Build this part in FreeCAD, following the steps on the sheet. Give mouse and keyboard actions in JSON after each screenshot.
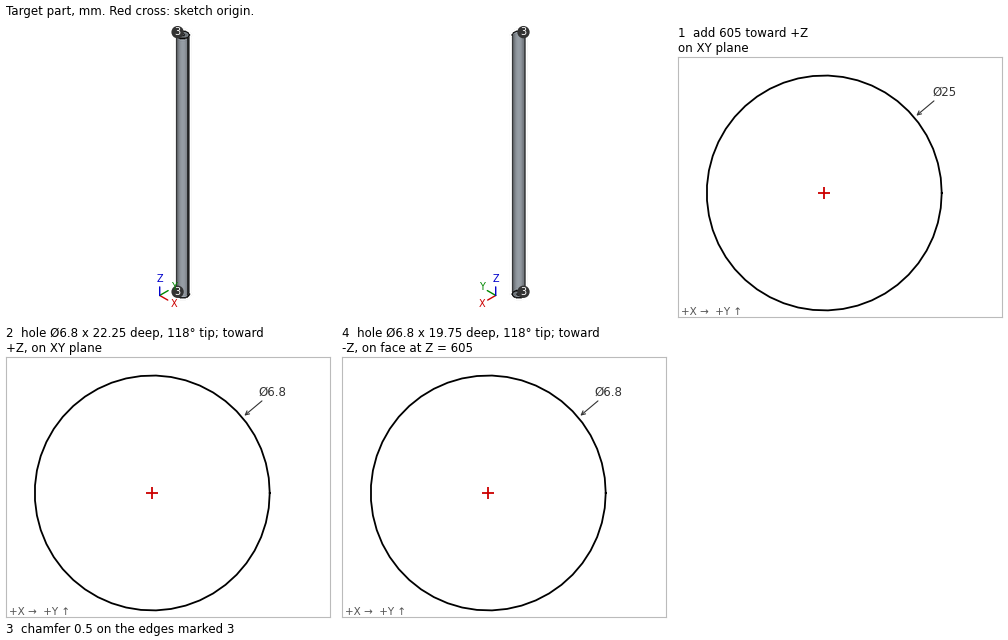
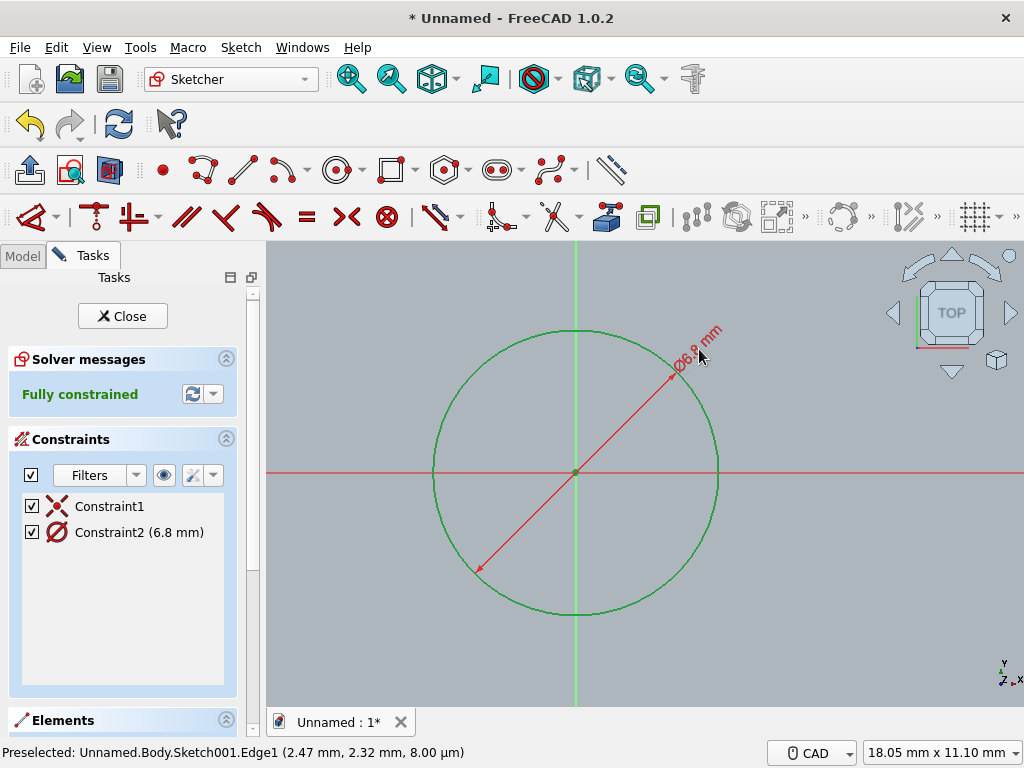
{"action": "left_click", "coordinate": [123, 316]}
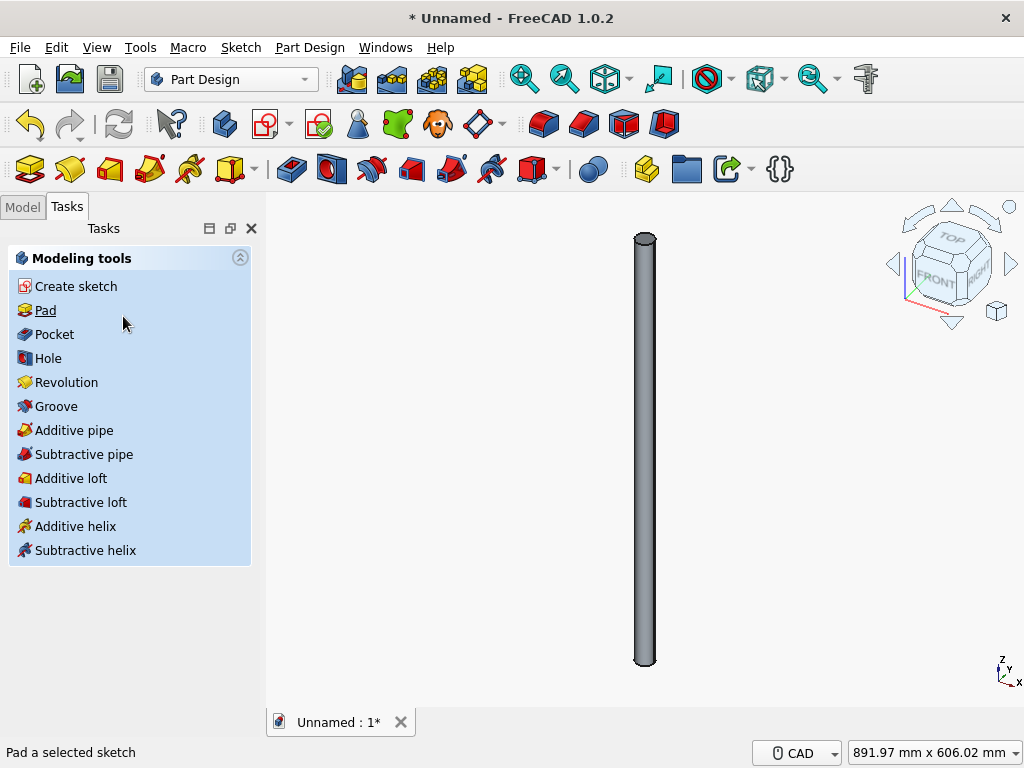
{"action": "left_click", "coordinate": [332, 170]}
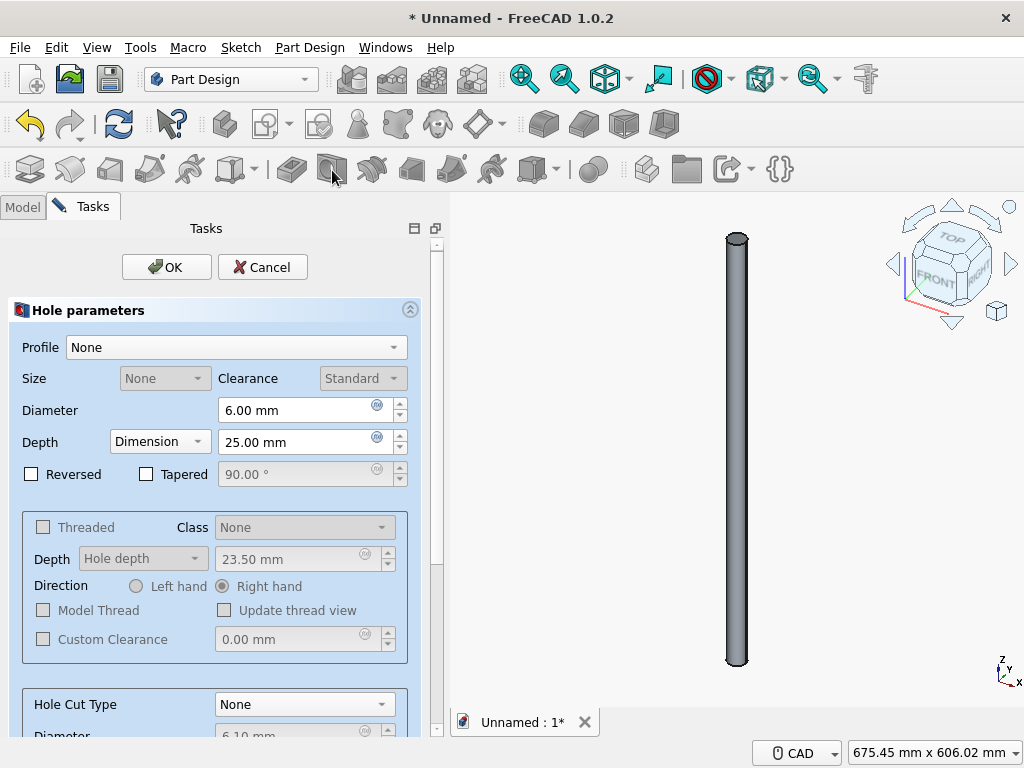
{"action": "triple_click", "coordinate": [305, 410]}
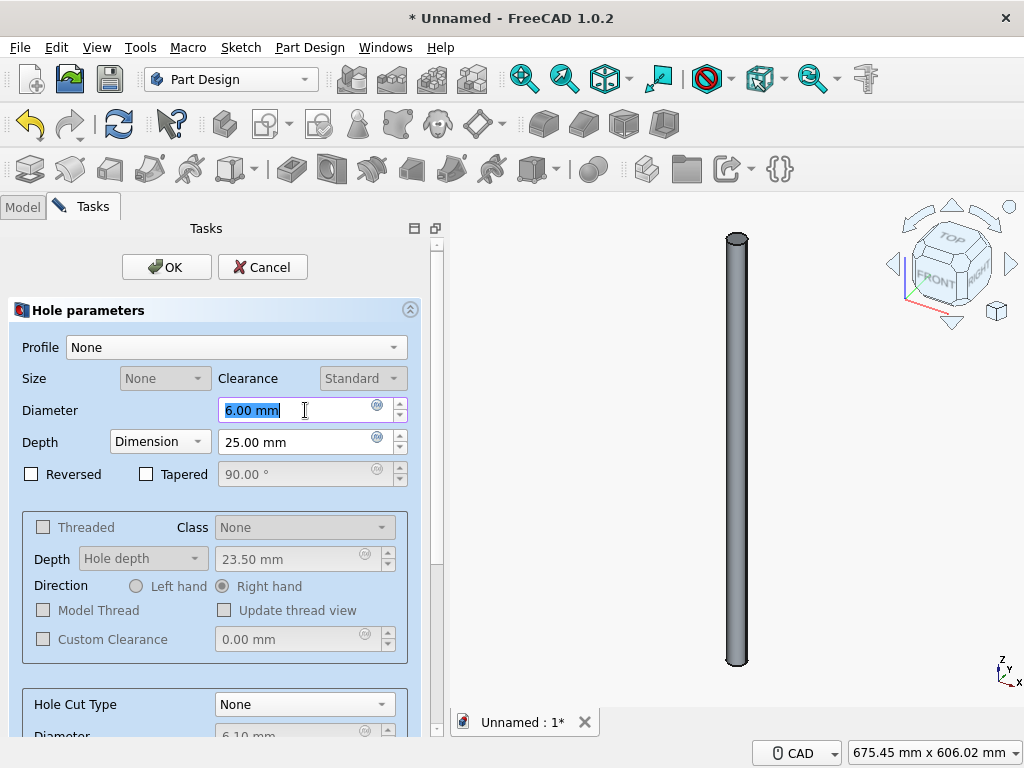
{"action": "type", "text": "6.8"}
{"action": "key", "text": "Tab"}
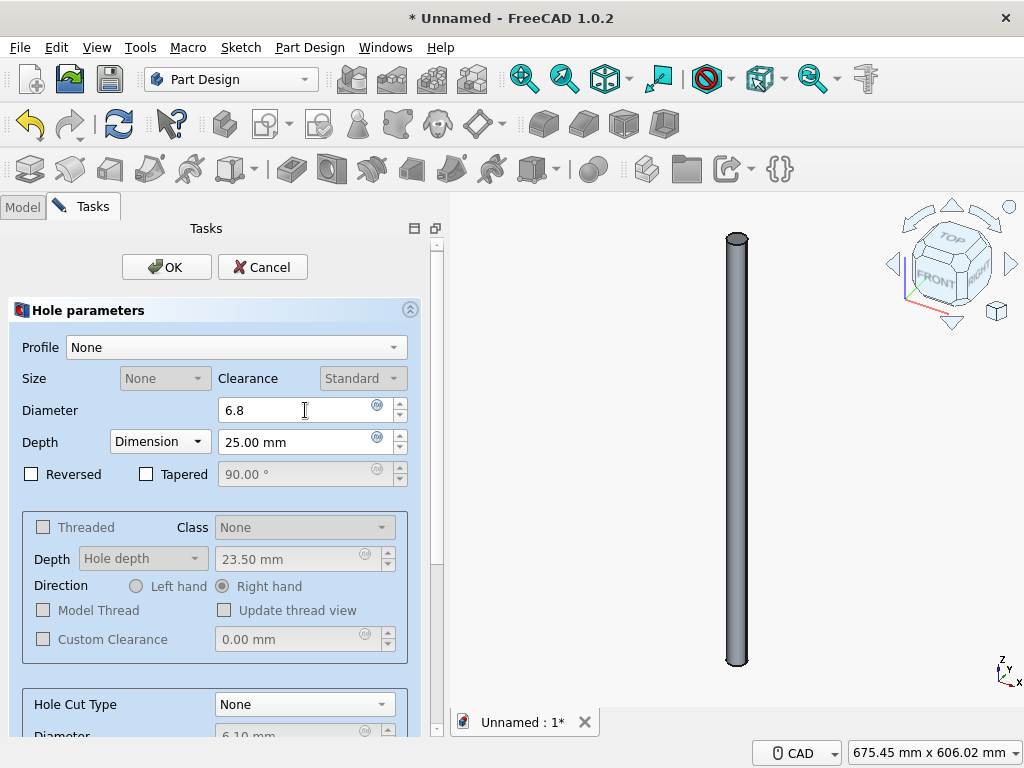
{"action": "triple_click", "coordinate": [305, 442]}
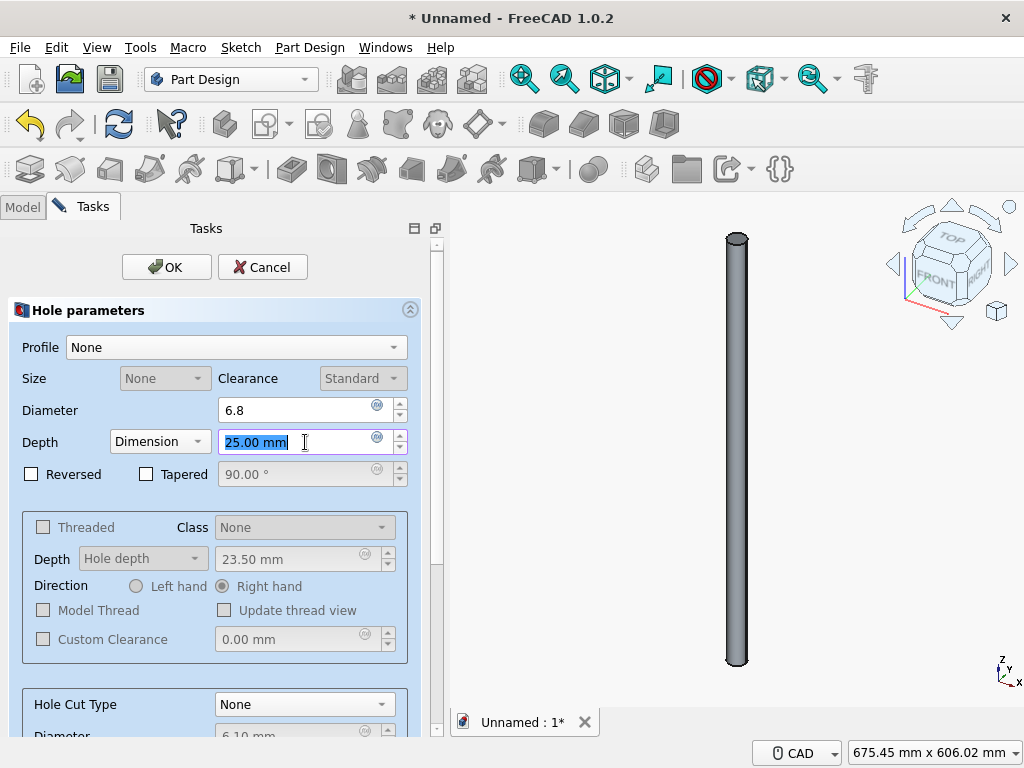
{"action": "type", "text": "22.25"}
{"action": "key", "text": "Tab"}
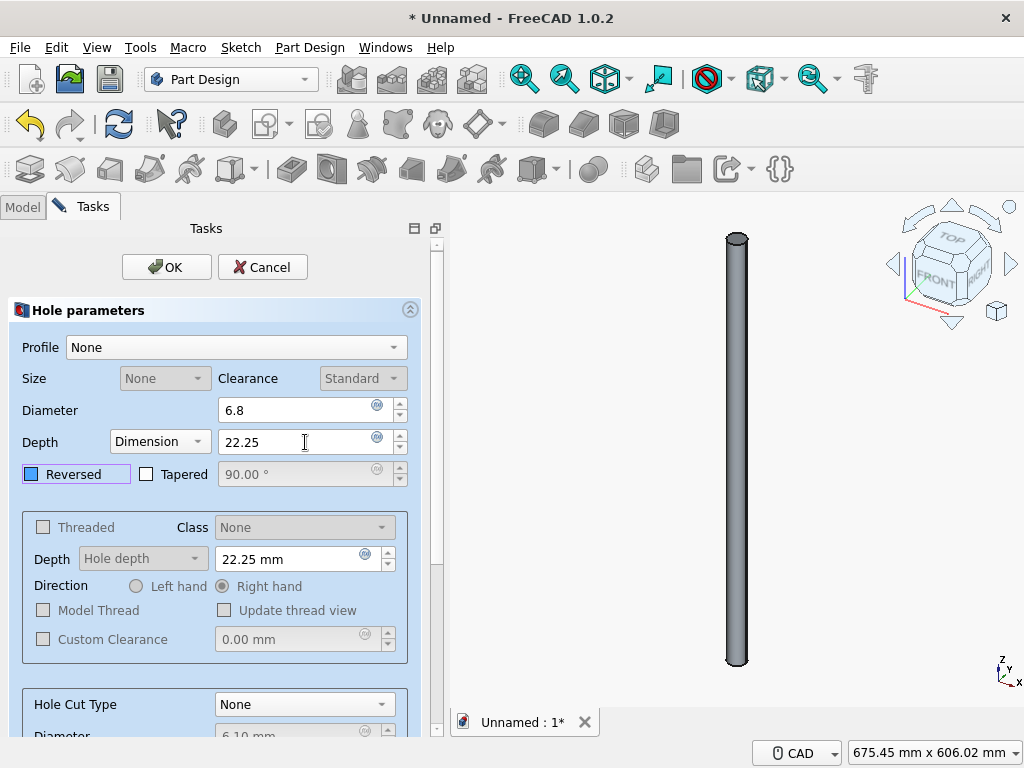
{"action": "left_click", "coordinate": [30, 474]}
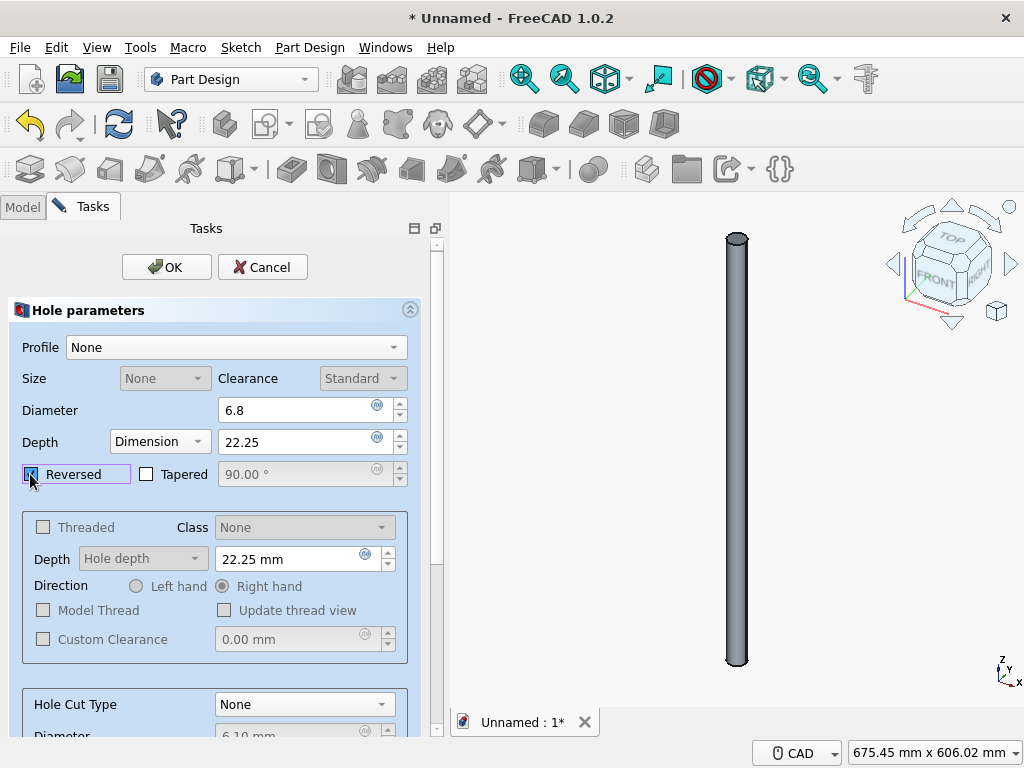
{"action": "left_click", "coordinate": [167, 267]}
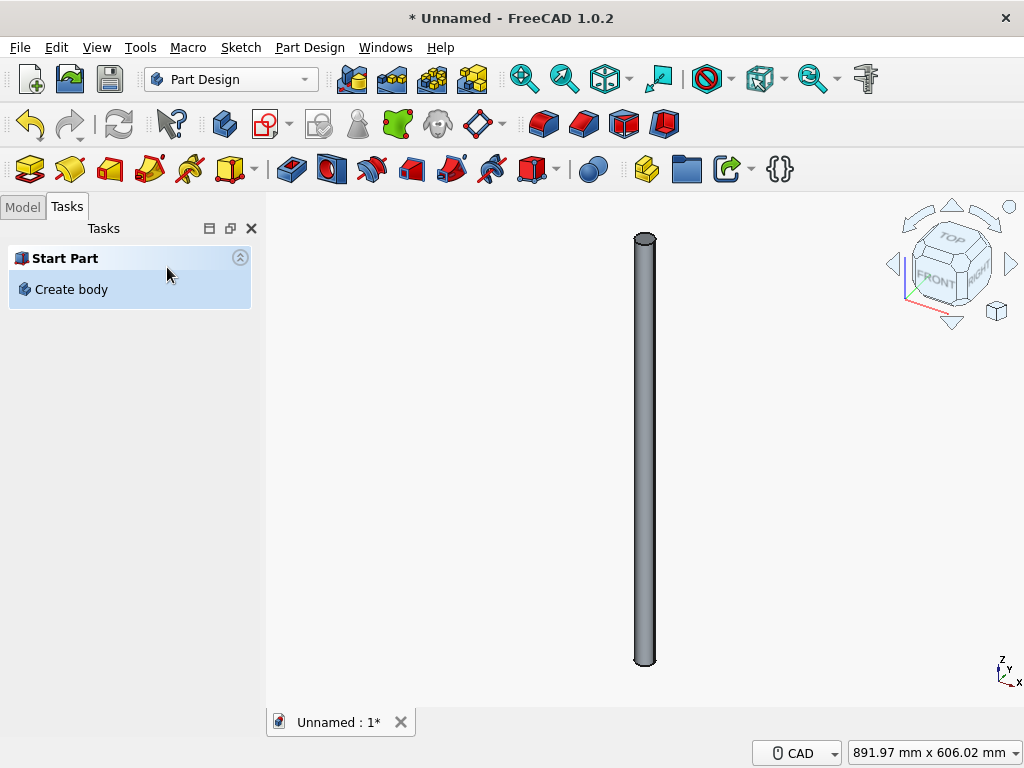
{"action": "left_click", "coordinate": [634, 660]}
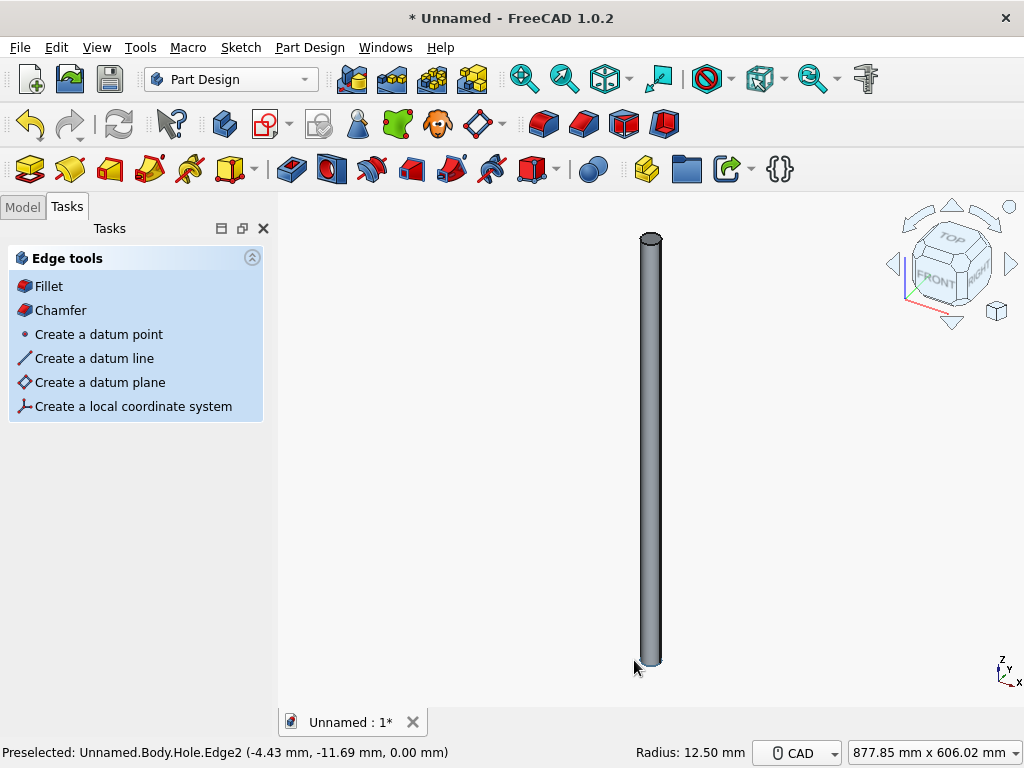
{"action": "left_click", "coordinate": [642, 235], "text": "ctrl"}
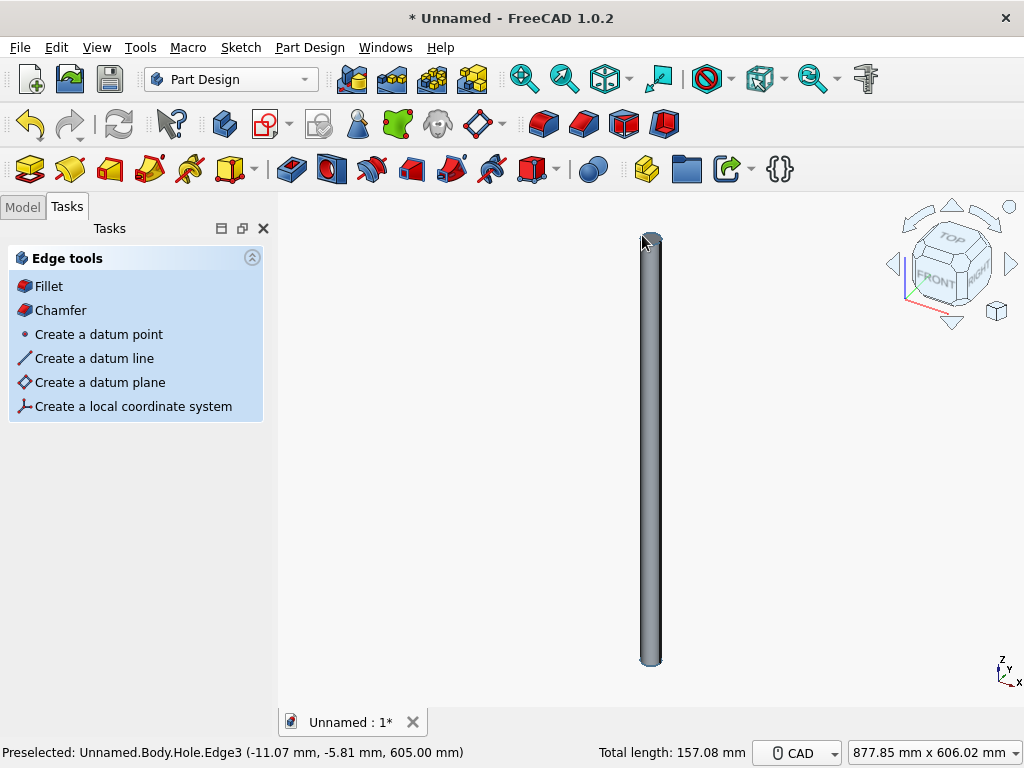
{"action": "left_click", "coordinate": [584, 124]}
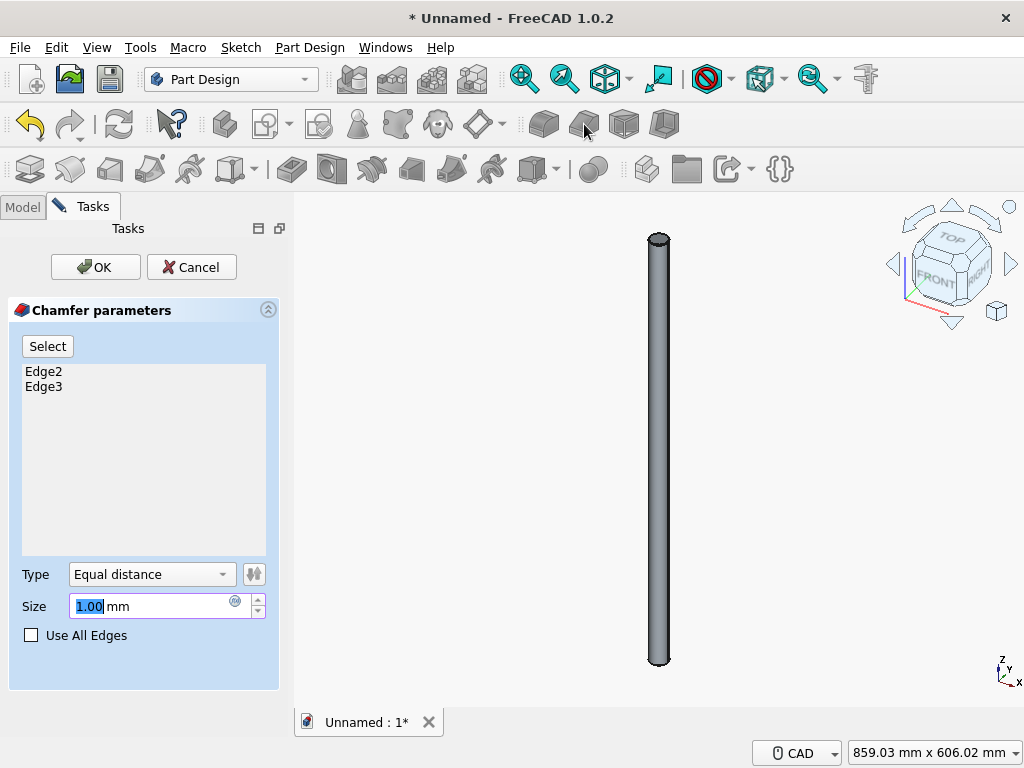
{"action": "type", "text": "0.5"}
{"action": "key", "text": "Tab"}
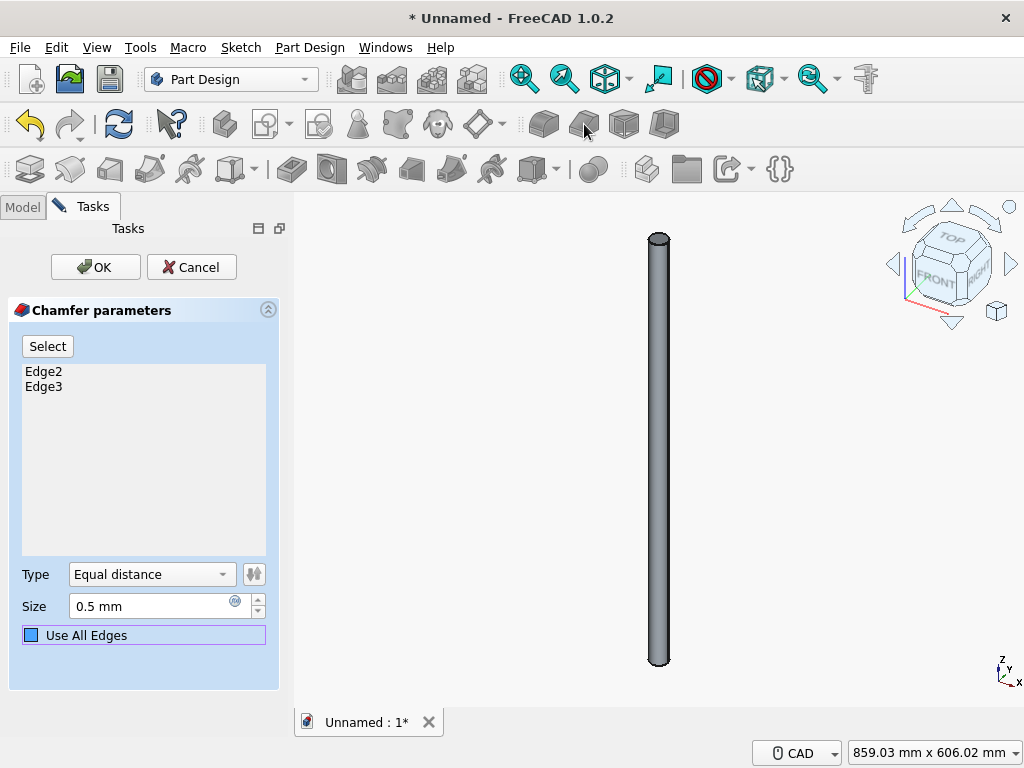
{"action": "left_click", "coordinate": [96, 267]}